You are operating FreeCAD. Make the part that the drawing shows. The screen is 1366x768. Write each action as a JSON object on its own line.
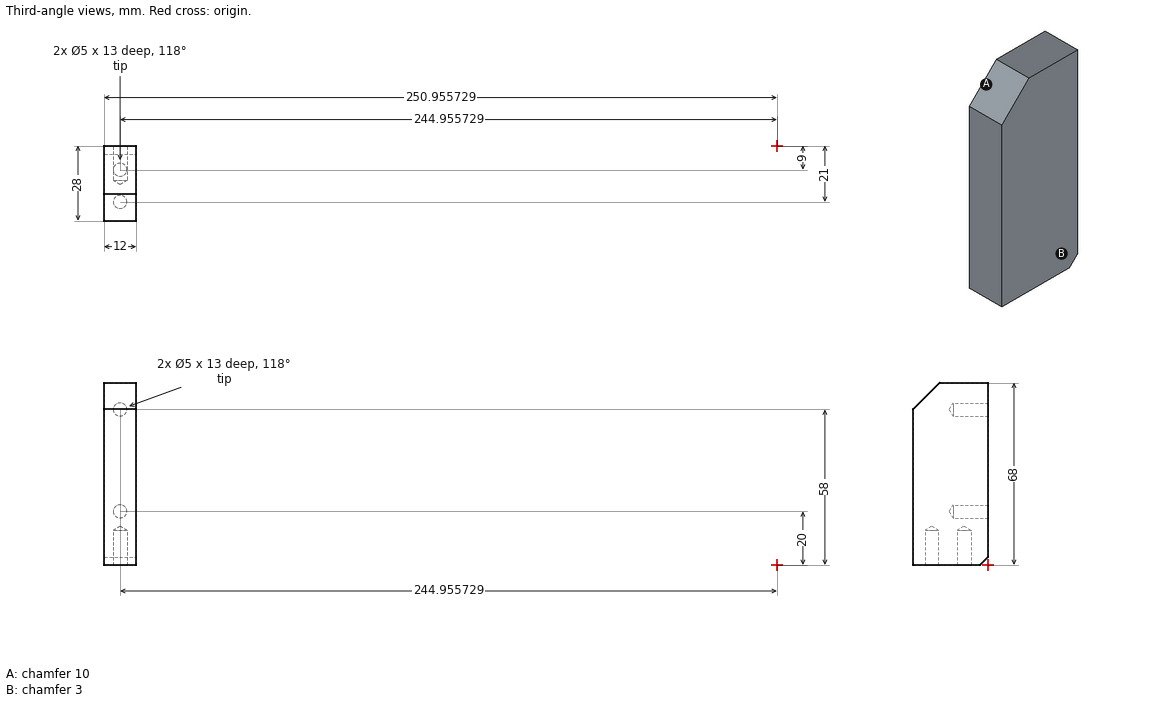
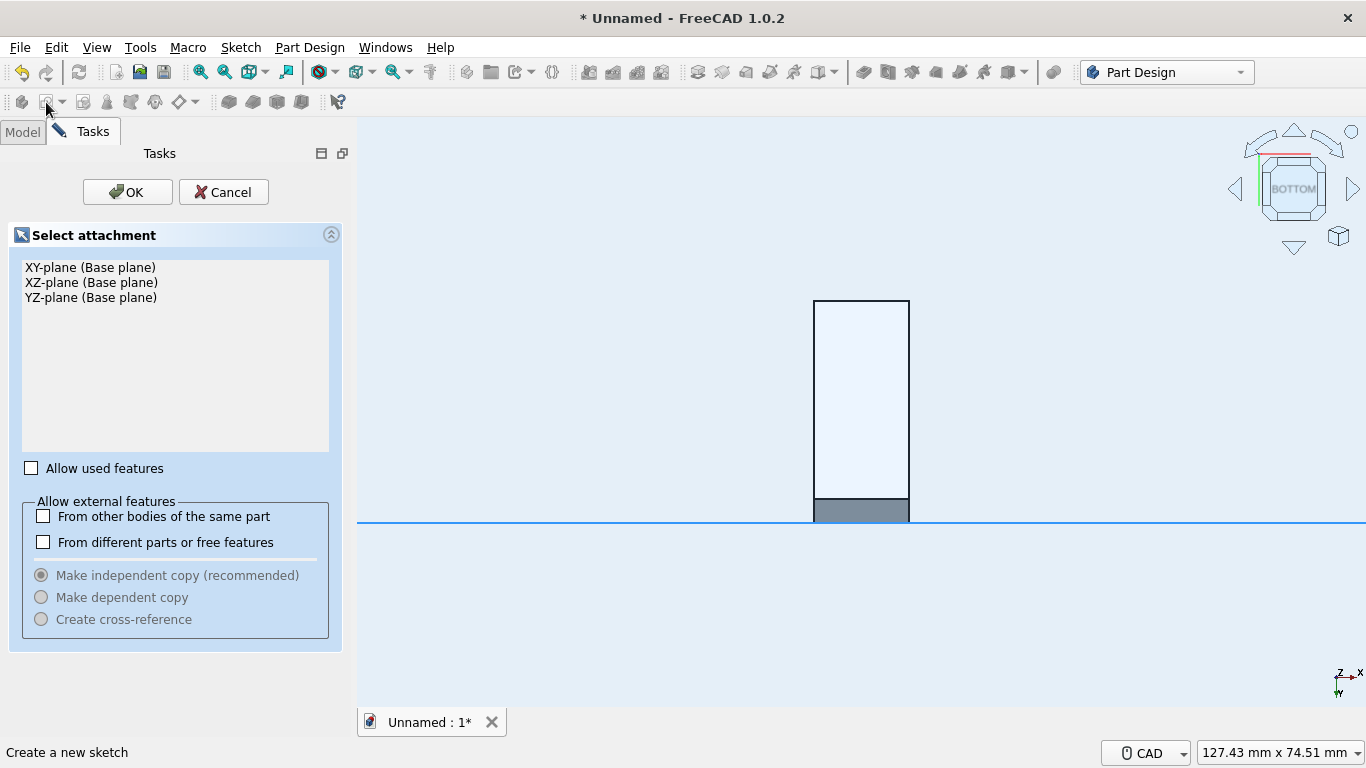
{"action": "left_click", "coordinate": [82, 268]}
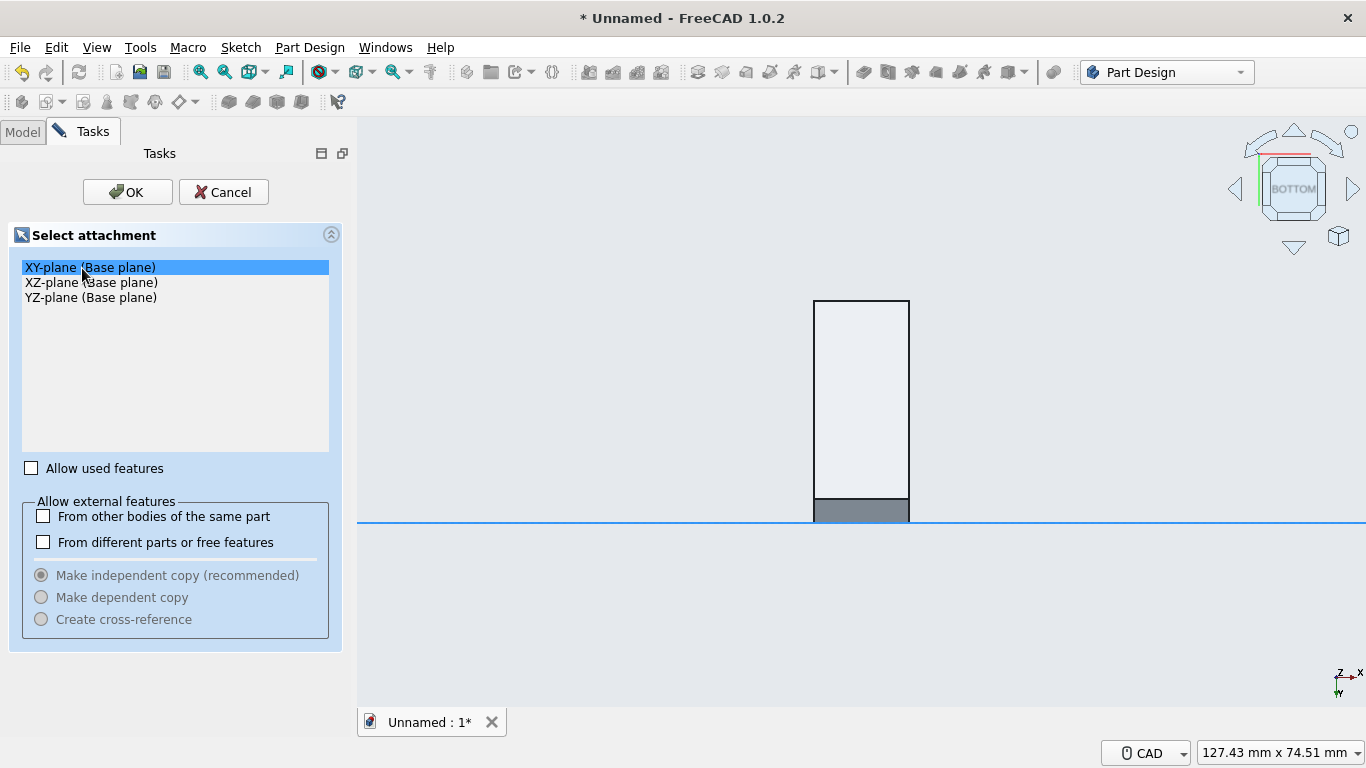
{"action": "left_click", "coordinate": [128, 192]}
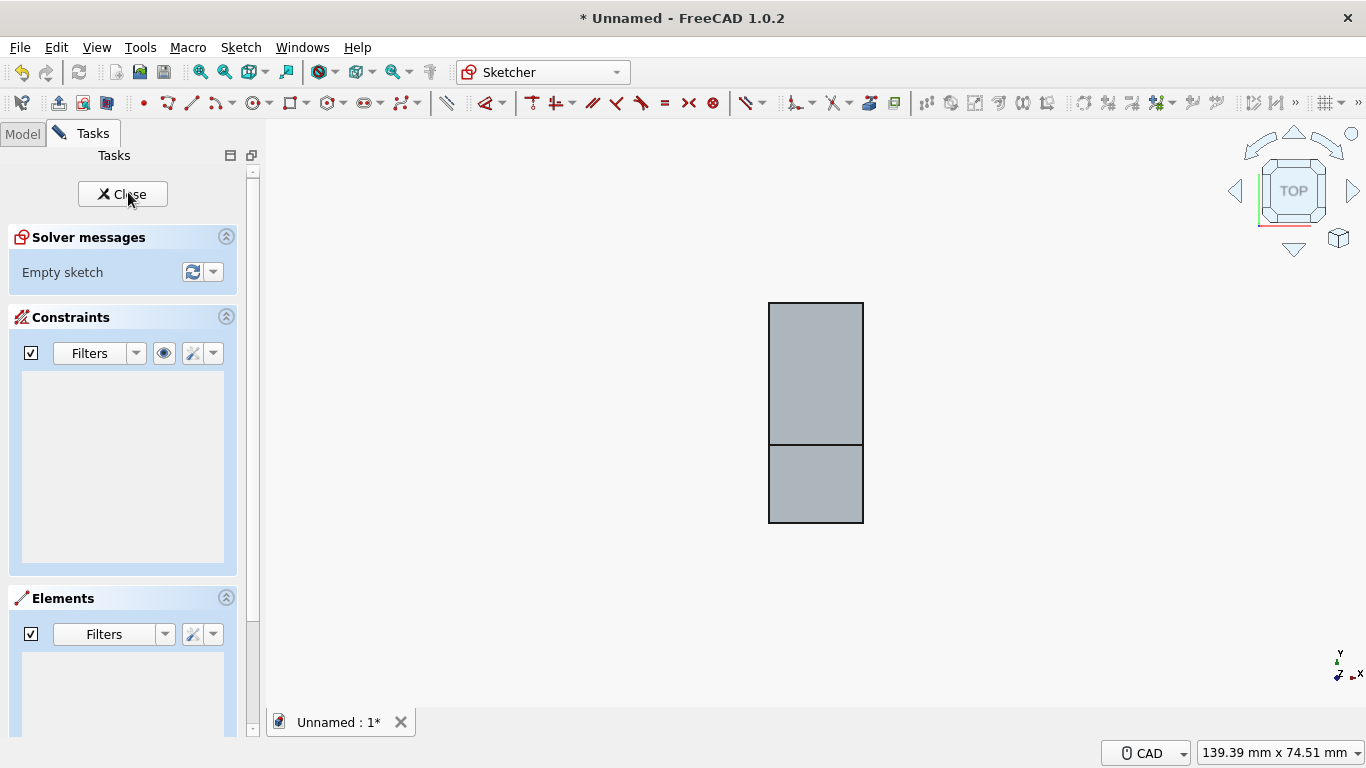
{"action": "left_click", "coordinate": [108, 104]}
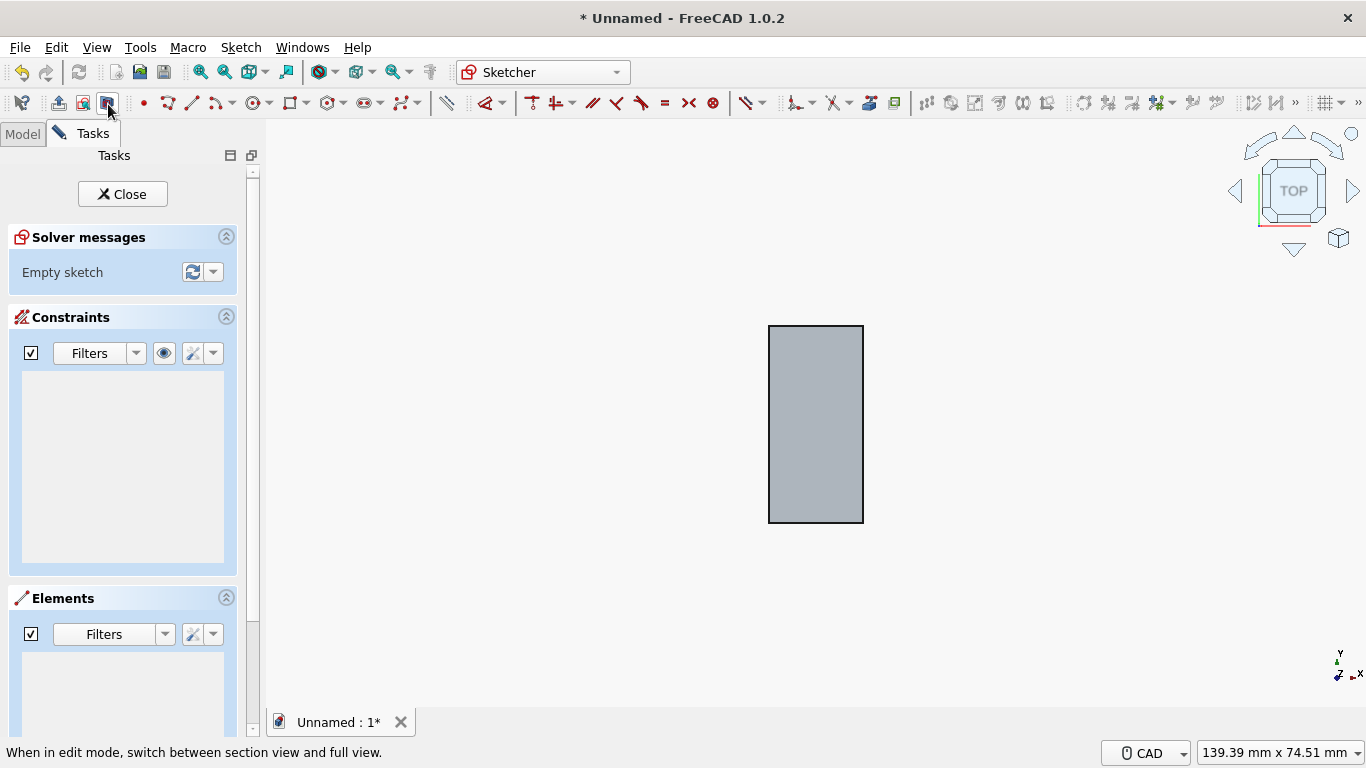
{"action": "scroll", "coordinate": [856, 425], "scroll_direction": "up", "scroll_amount": 5}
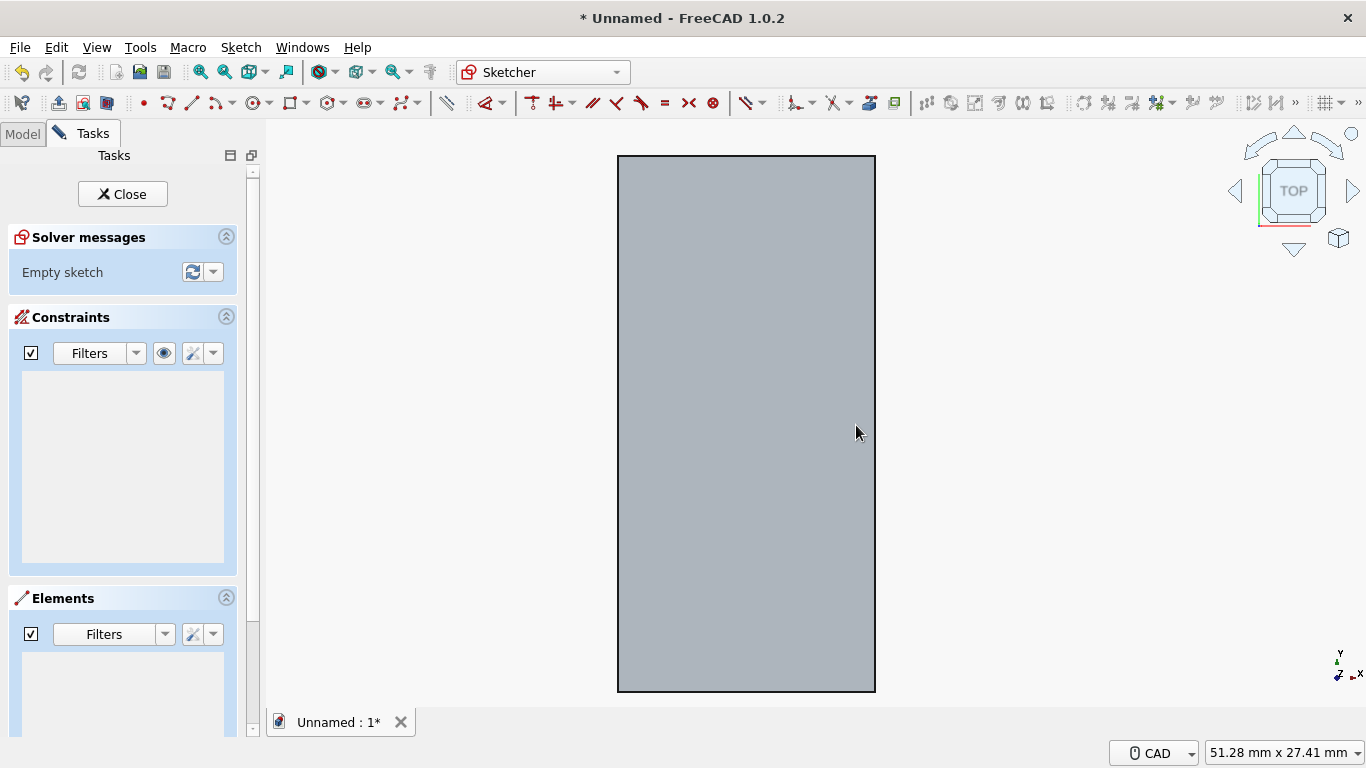
{"action": "left_click", "coordinate": [254, 104]}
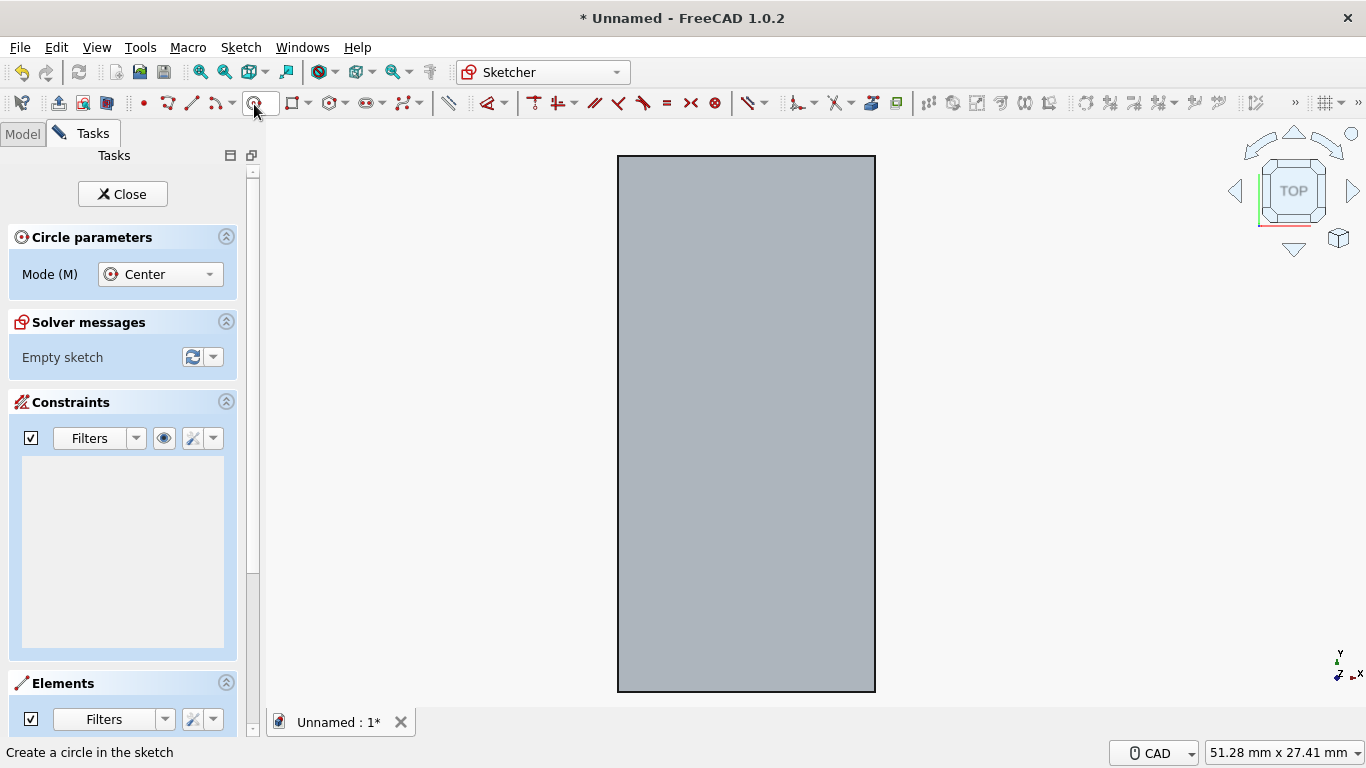
{"action": "left_click", "coordinate": [746, 284]}
{"action": "mouse_move", "coordinate": [784, 246]}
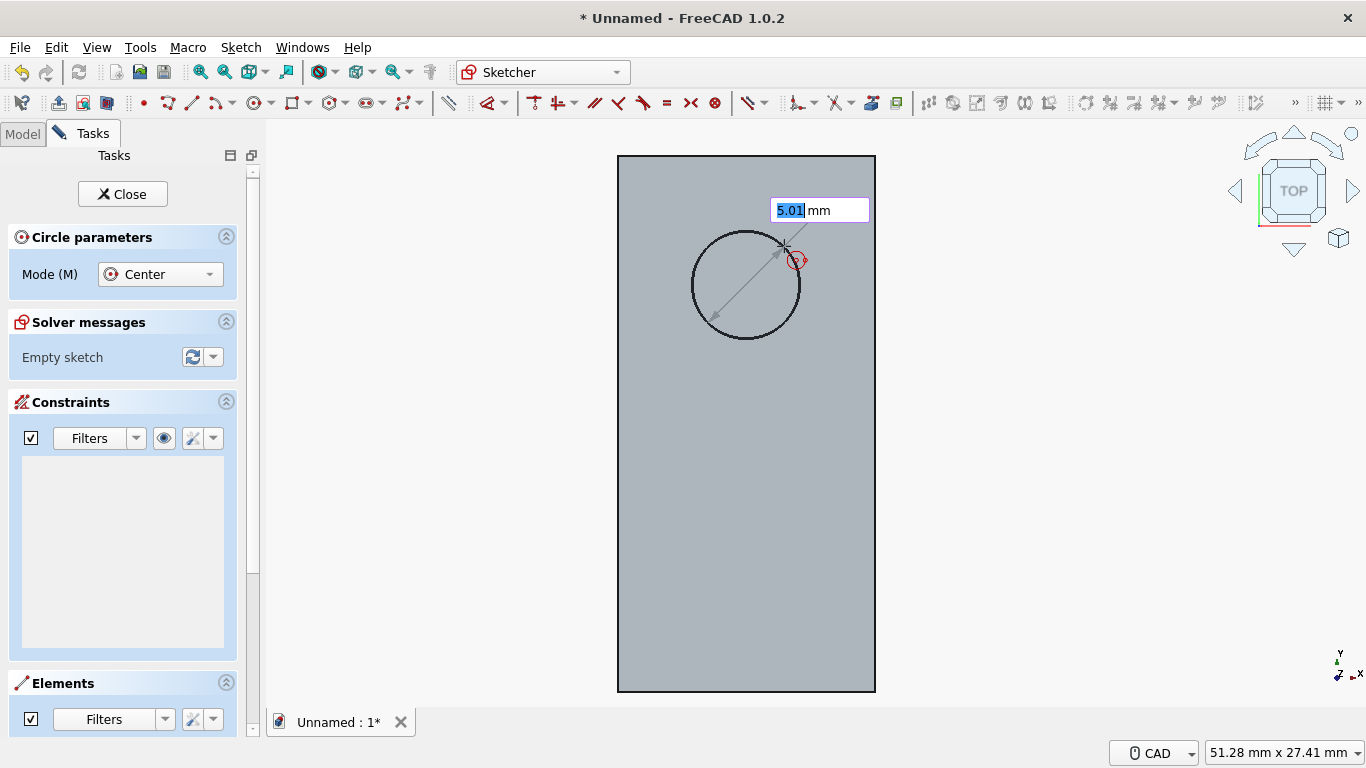
{"action": "type", "text": "5"}
{"action": "key", "text": "Return"}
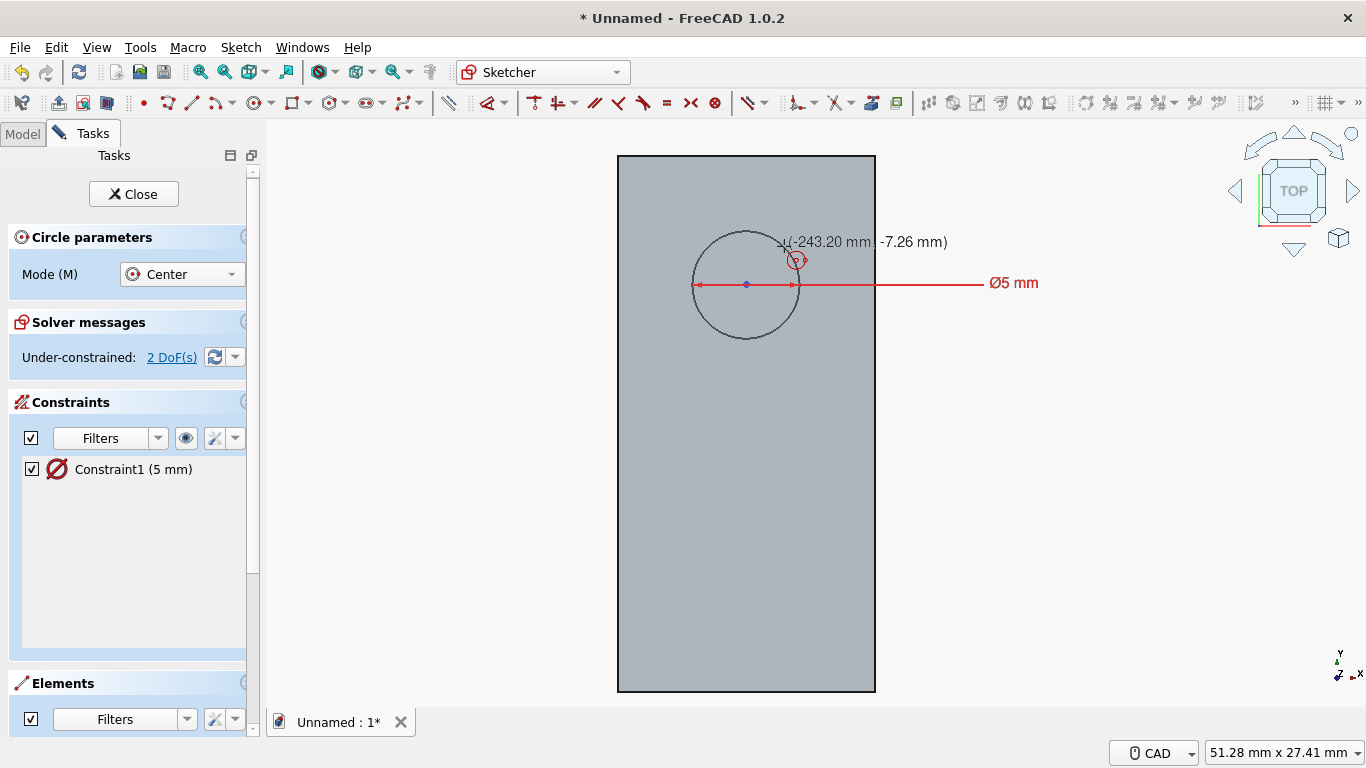
{"action": "left_click", "coordinate": [746, 542]}
{"action": "mouse_move", "coordinate": [784, 504]}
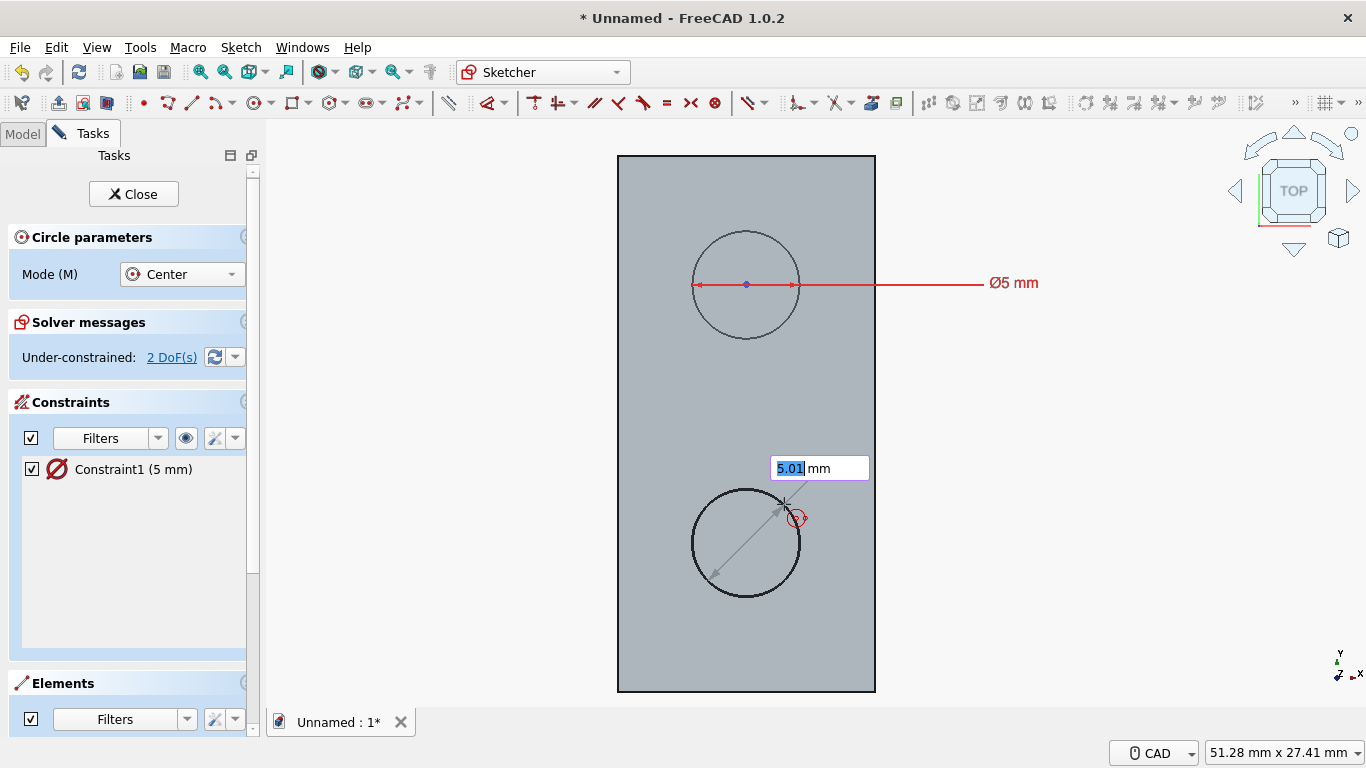
{"action": "type", "text": "5"}
{"action": "key", "text": "Return"}
{"action": "key", "text": "Escape"}